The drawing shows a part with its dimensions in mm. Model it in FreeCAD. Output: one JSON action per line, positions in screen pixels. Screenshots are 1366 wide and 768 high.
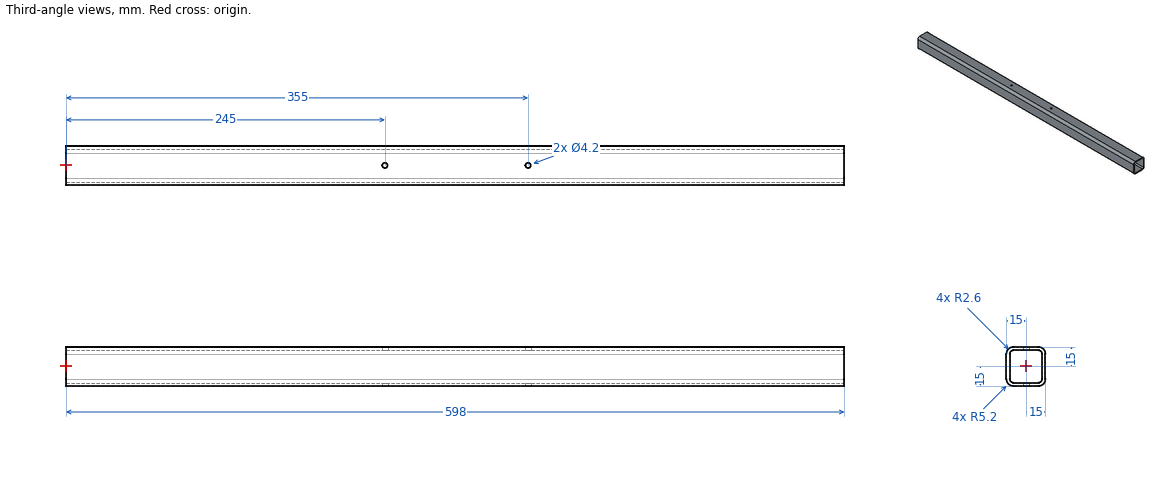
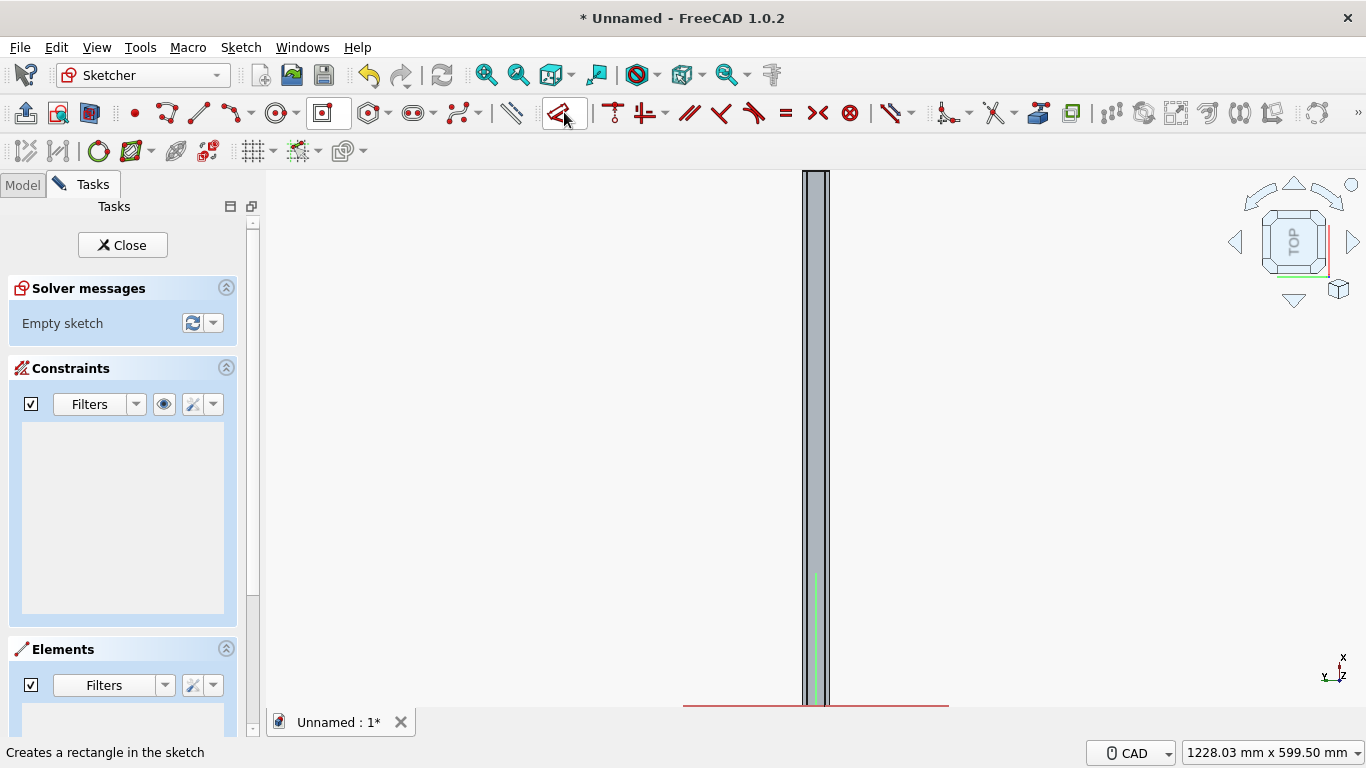
{"action": "scroll", "coordinate": [846, 437], "scroll_direction": "up", "scroll_amount": 6}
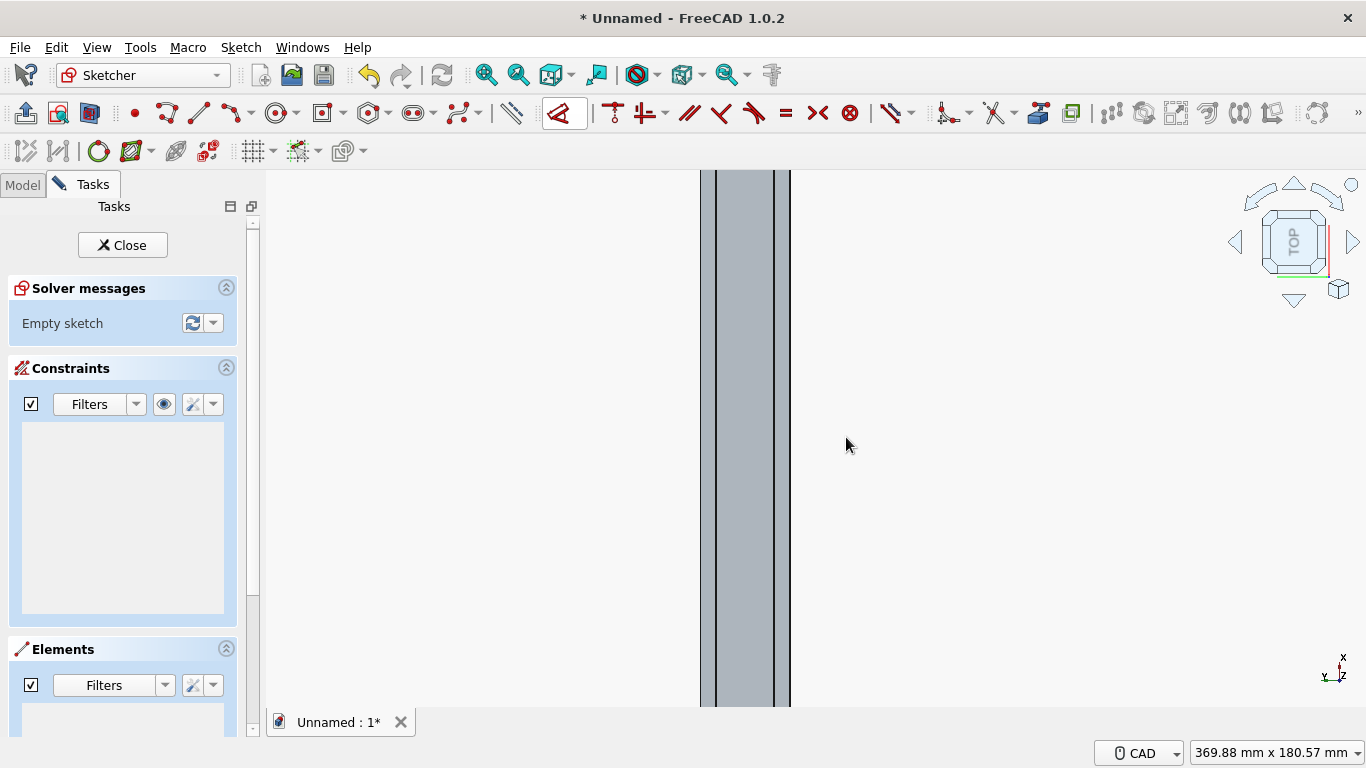
{"action": "left_click", "coordinate": [276, 114]}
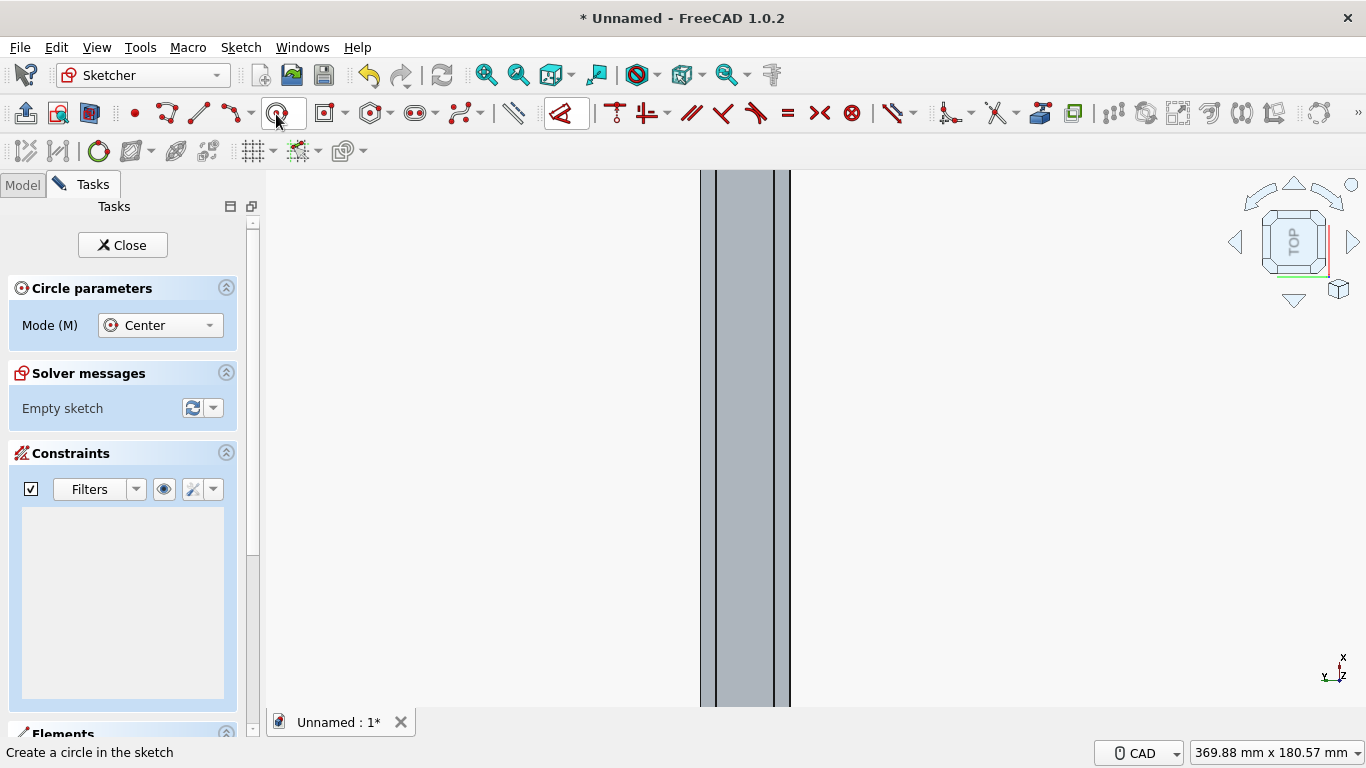
{"action": "scroll", "coordinate": [745, 274], "scroll_direction": "up", "scroll_amount": 7}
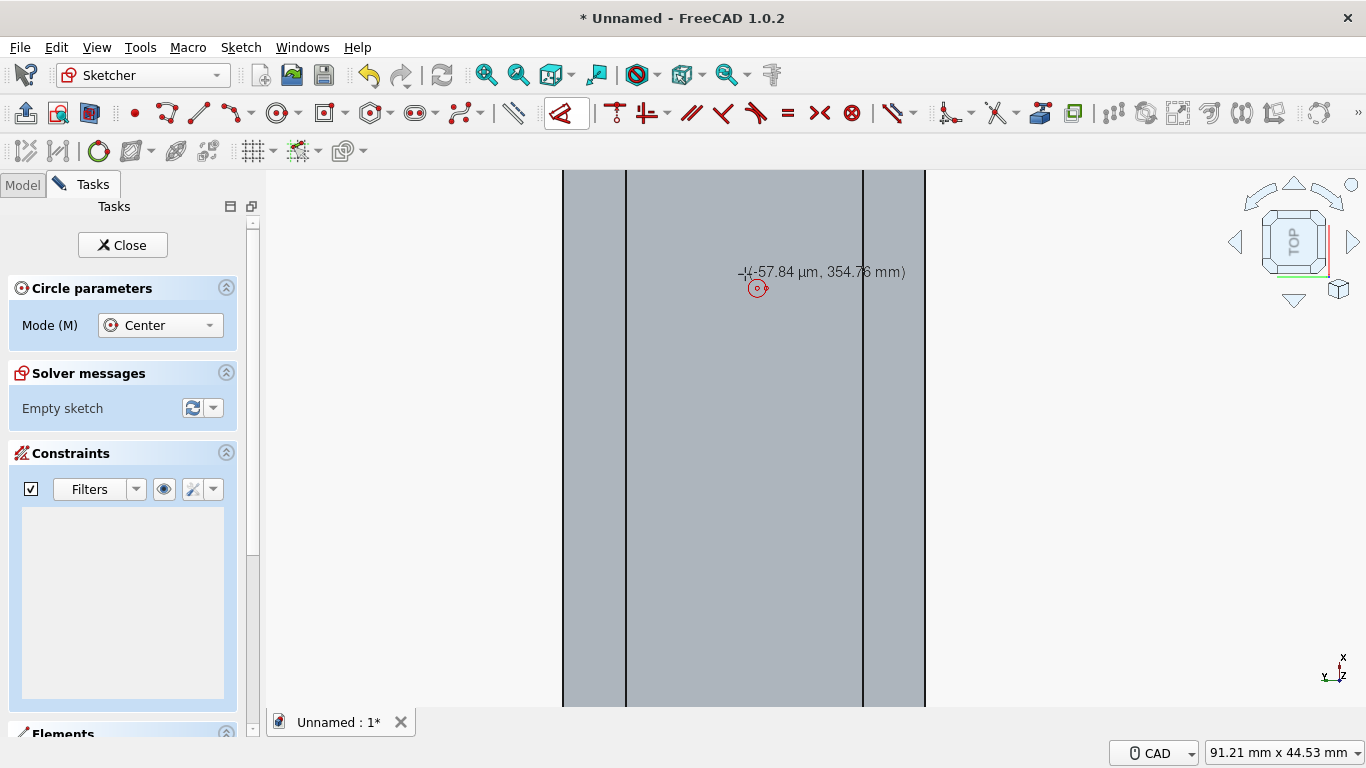
{"action": "scroll", "coordinate": [749, 275], "scroll_direction": "down", "scroll_amount": 7}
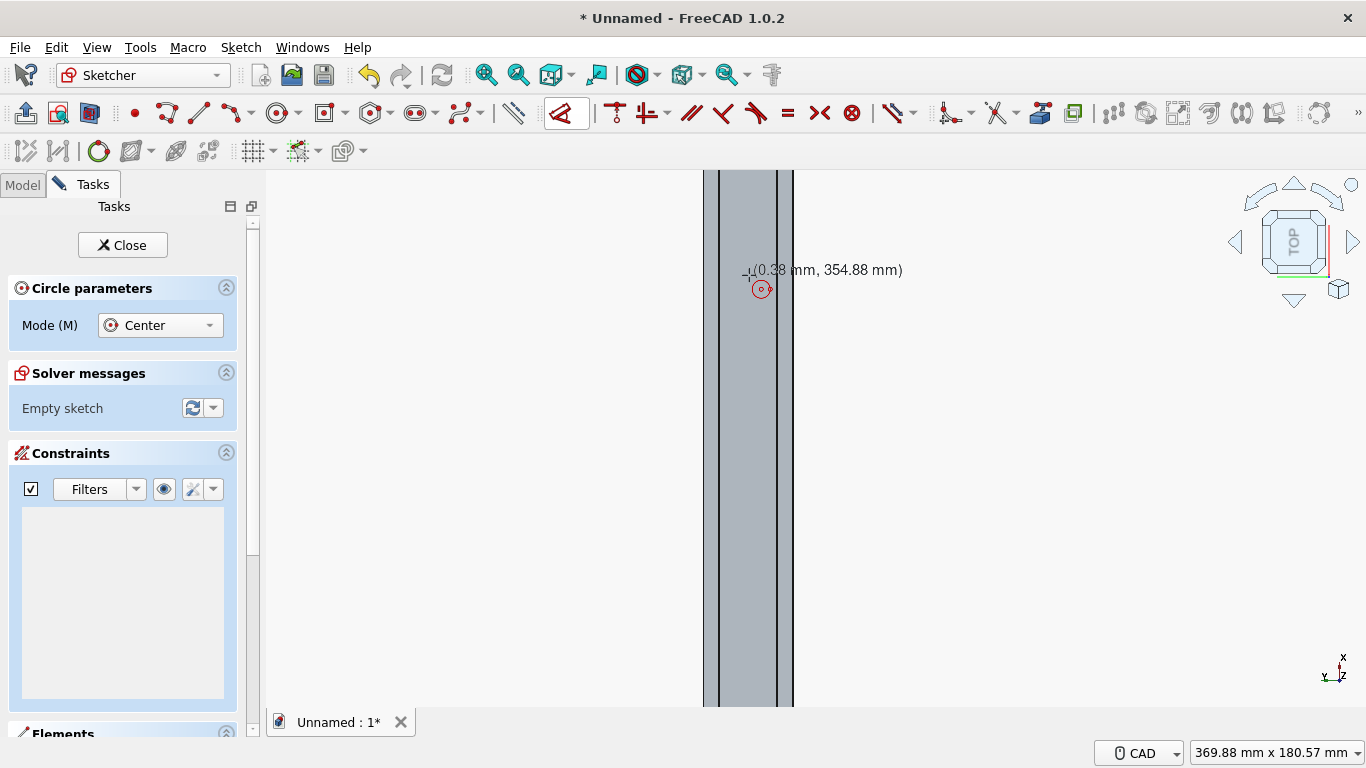
{"action": "left_click", "coordinate": [748, 275]}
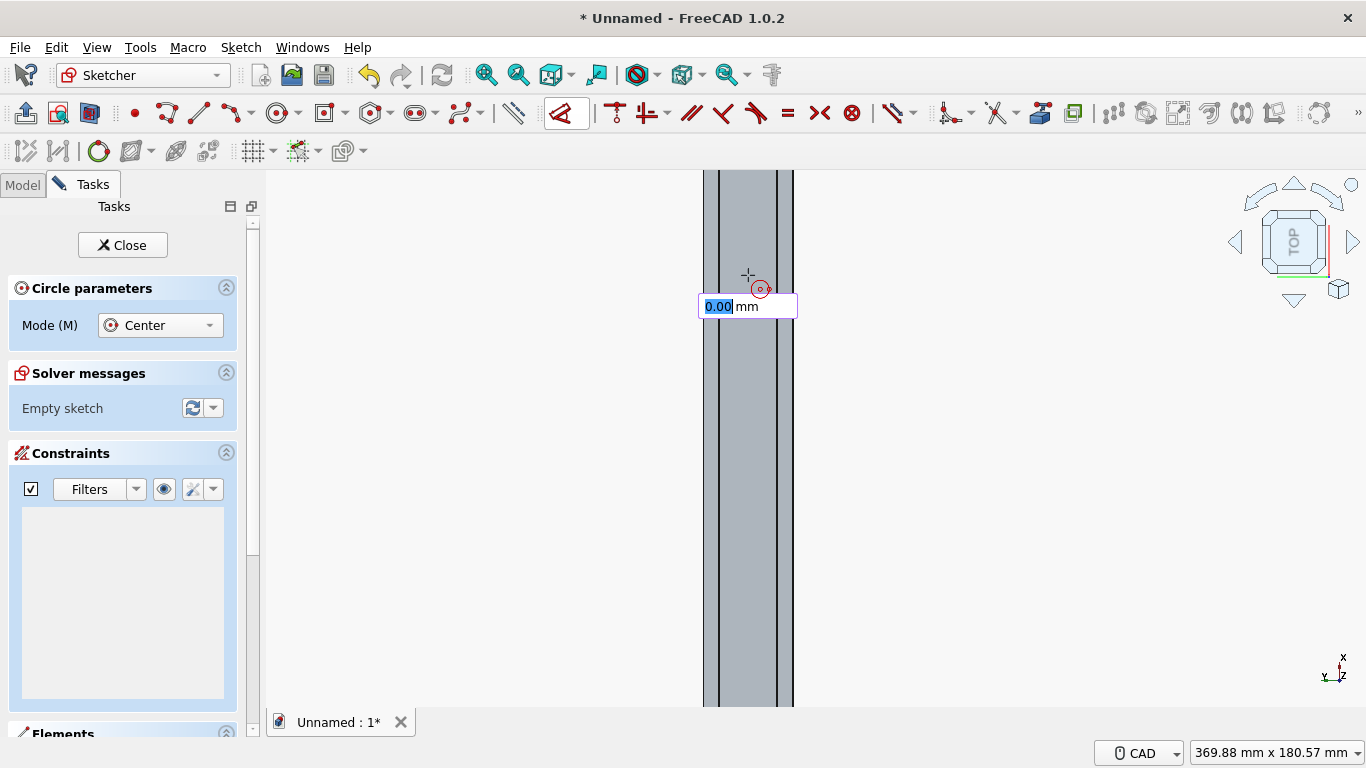
{"action": "scroll", "coordinate": [754, 273], "scroll_direction": "up", "scroll_amount": 5}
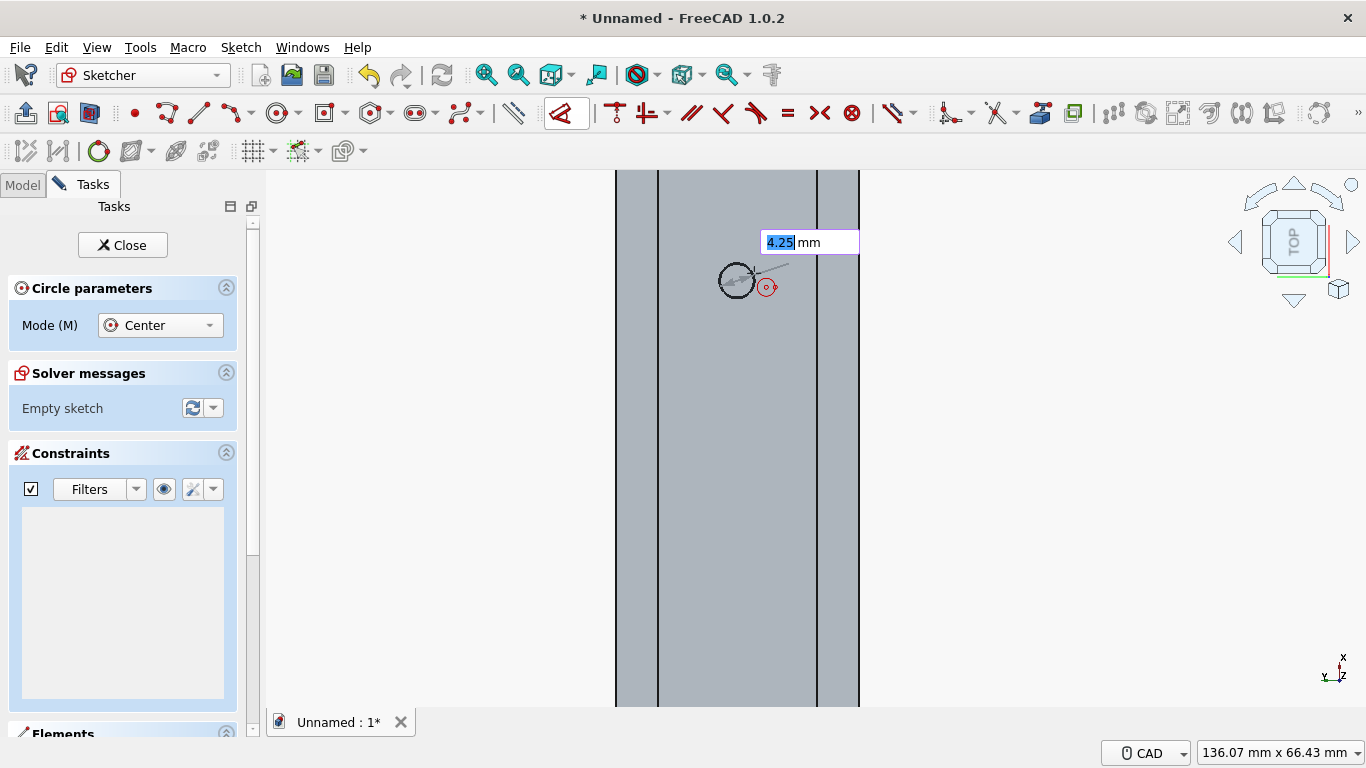
{"action": "left_click", "coordinate": [753, 272]}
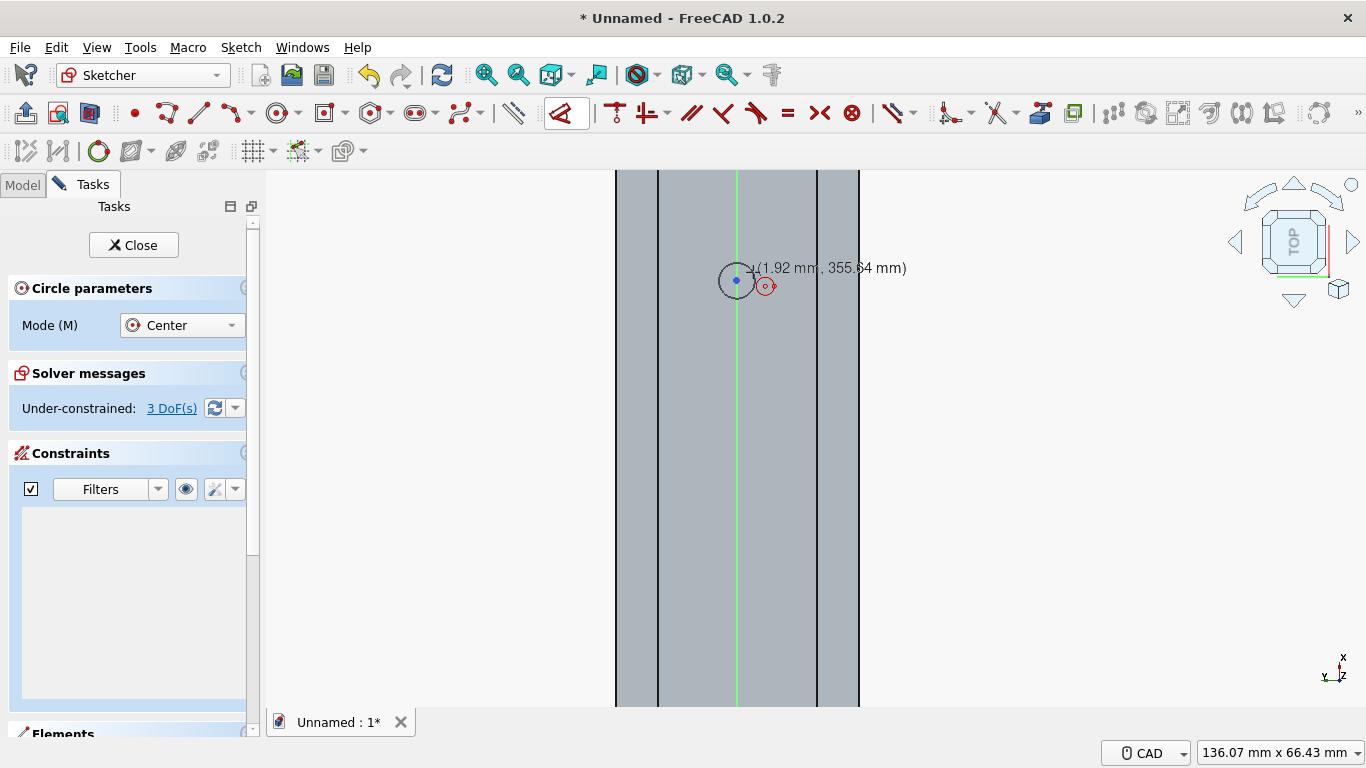
{"action": "scroll", "coordinate": [753, 273], "scroll_direction": "down", "scroll_amount": 5}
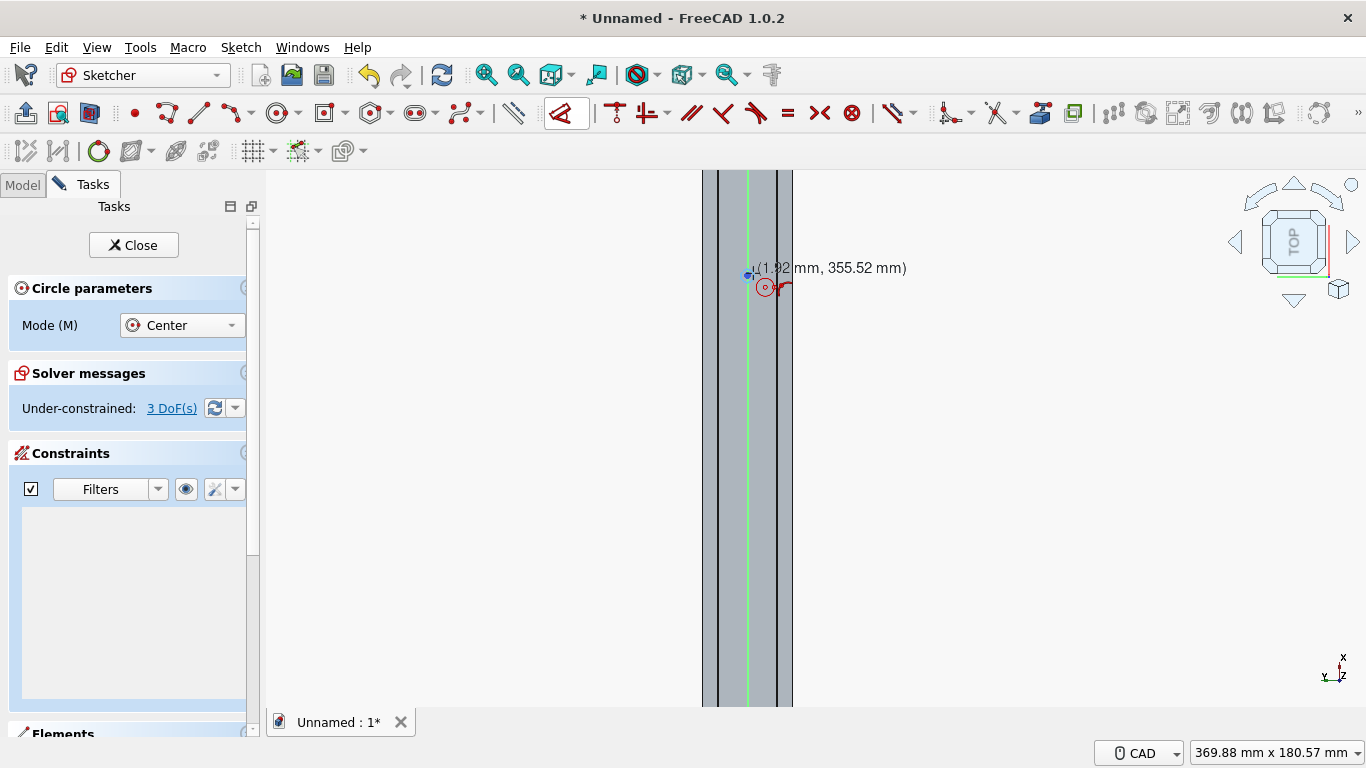
{"action": "scroll", "coordinate": [748, 602], "scroll_direction": "up", "scroll_amount": 7}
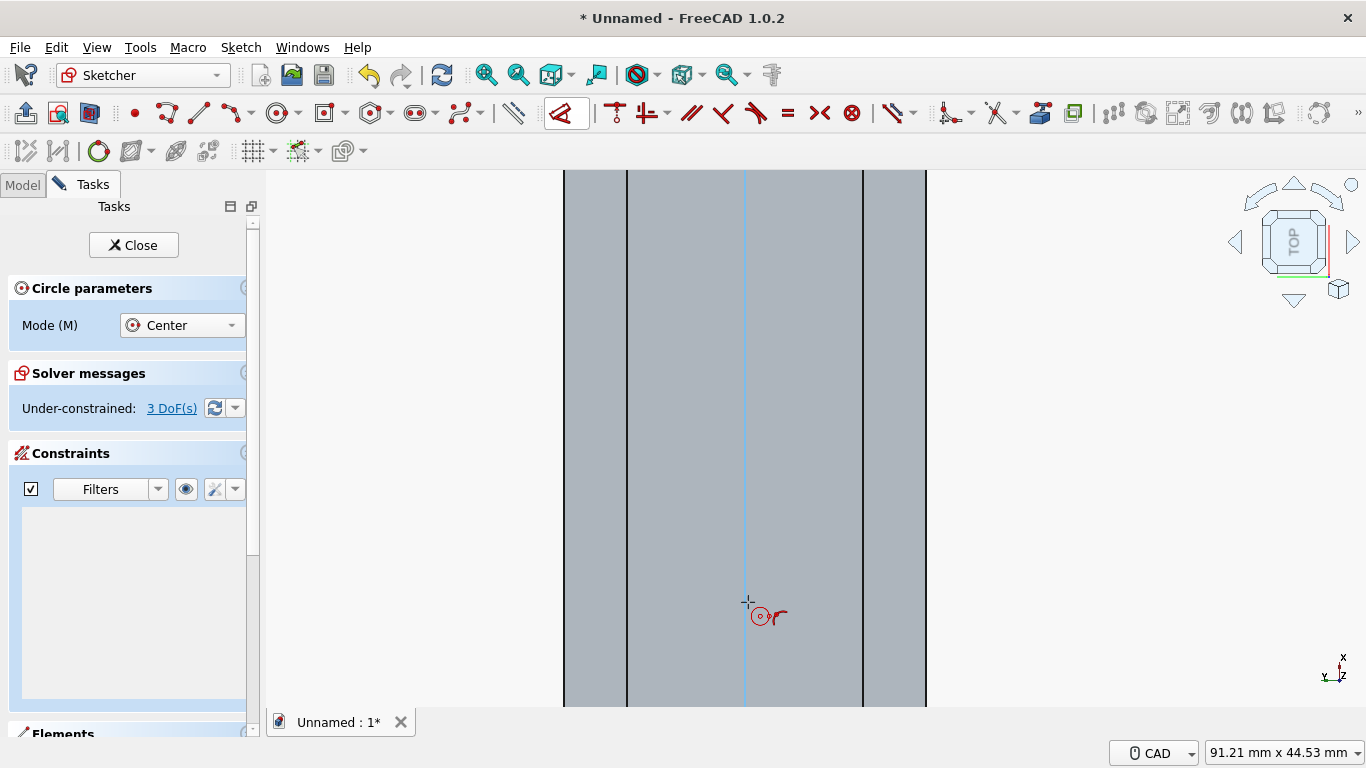
{"action": "scroll", "coordinate": [748, 603], "scroll_direction": "down", "scroll_amount": 7}